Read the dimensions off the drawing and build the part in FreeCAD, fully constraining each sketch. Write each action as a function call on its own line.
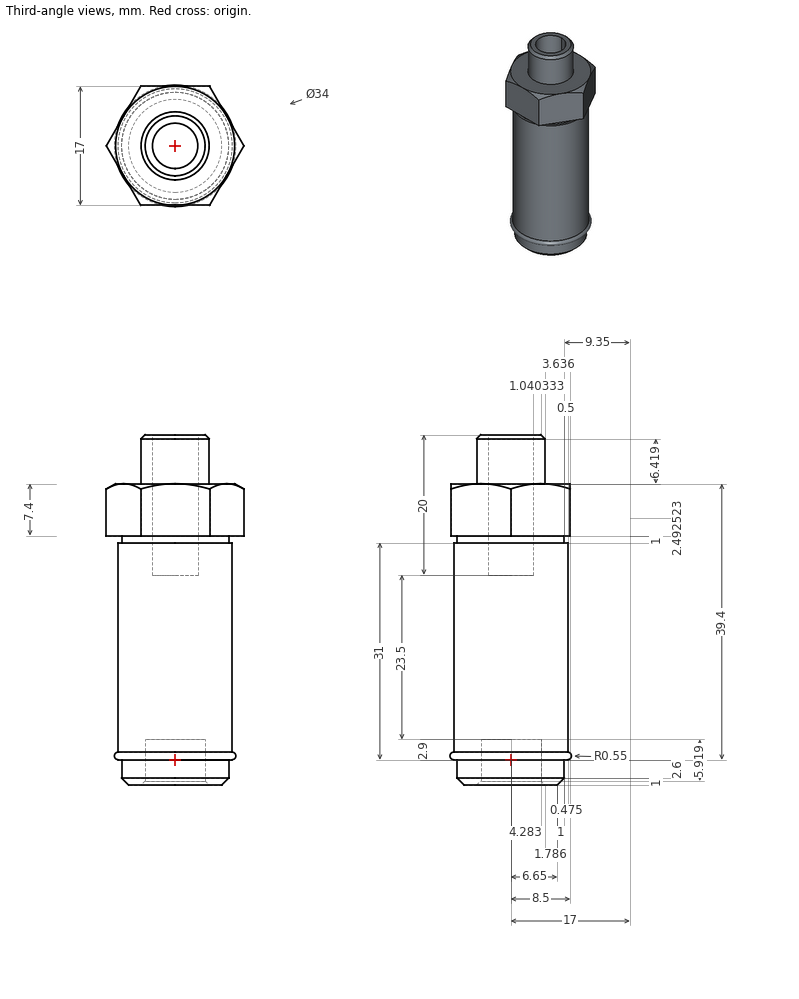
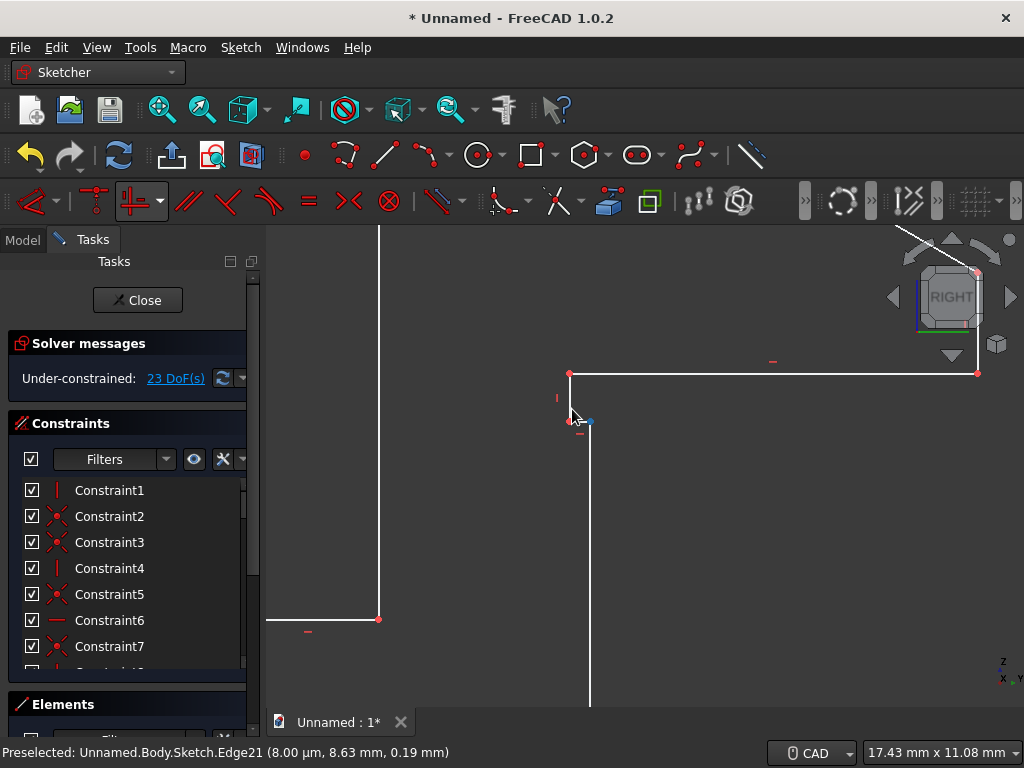
click(570, 407)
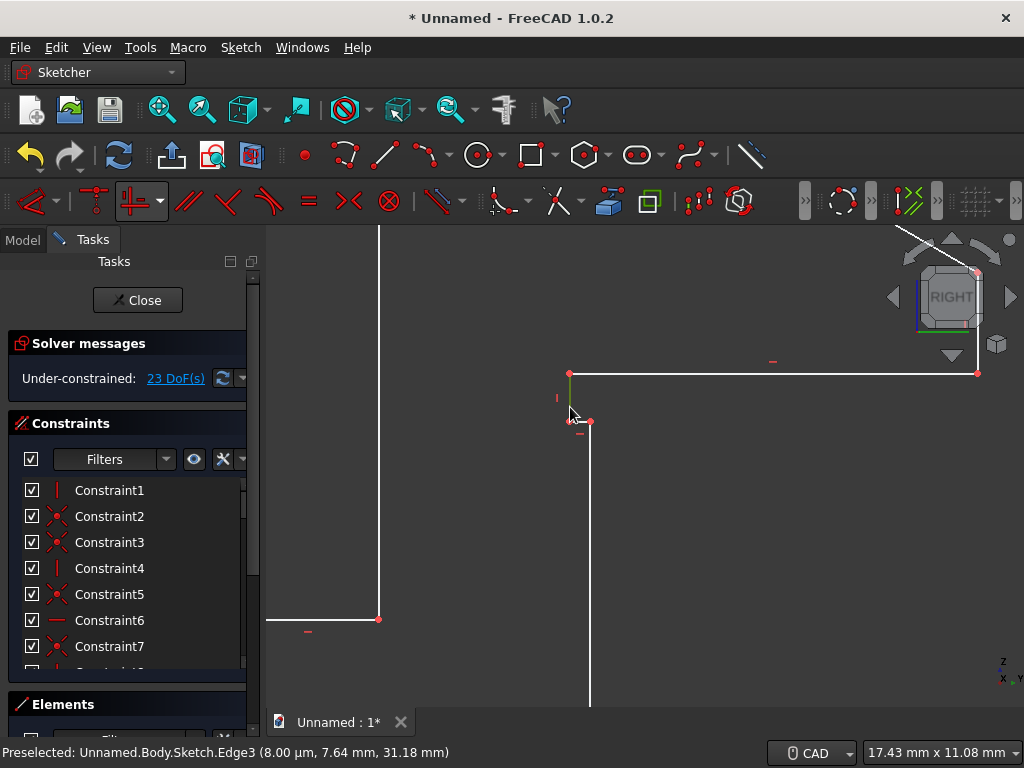
key(i)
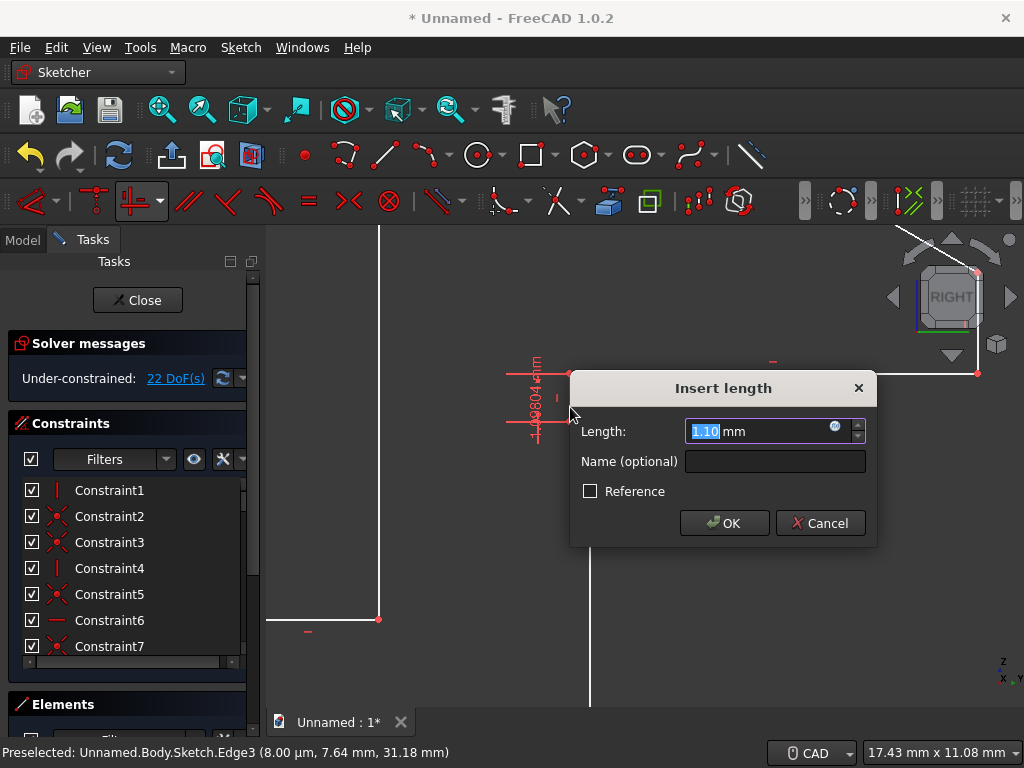
text(1)
key(Return)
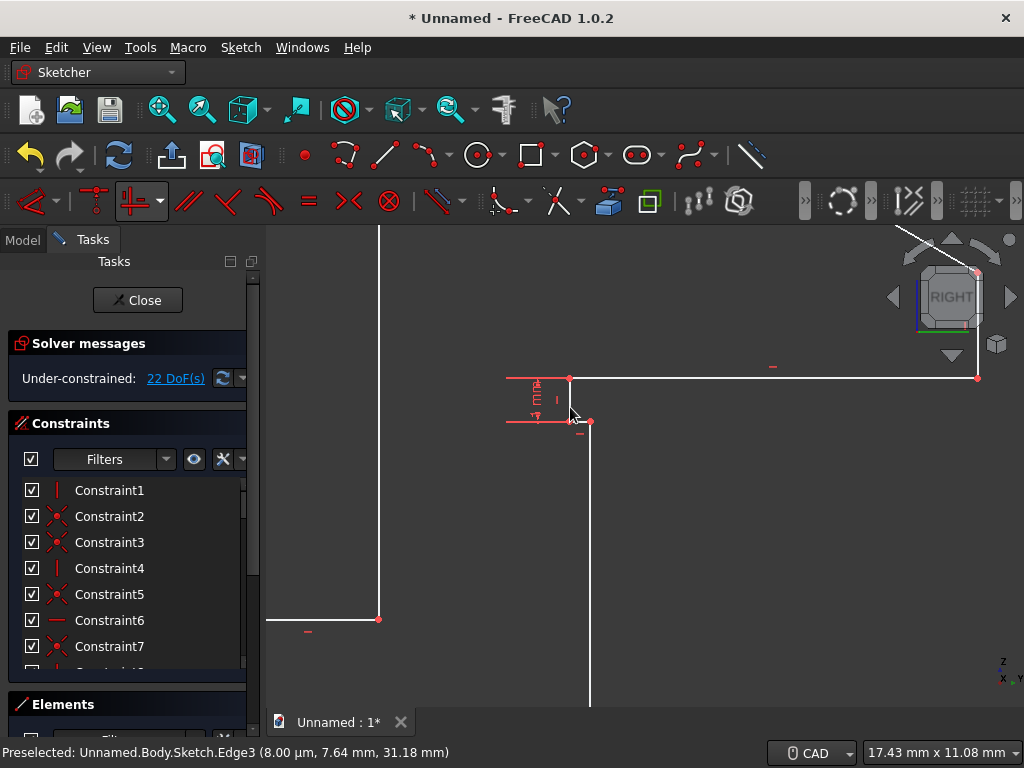
scroll(572, 408, down, 10)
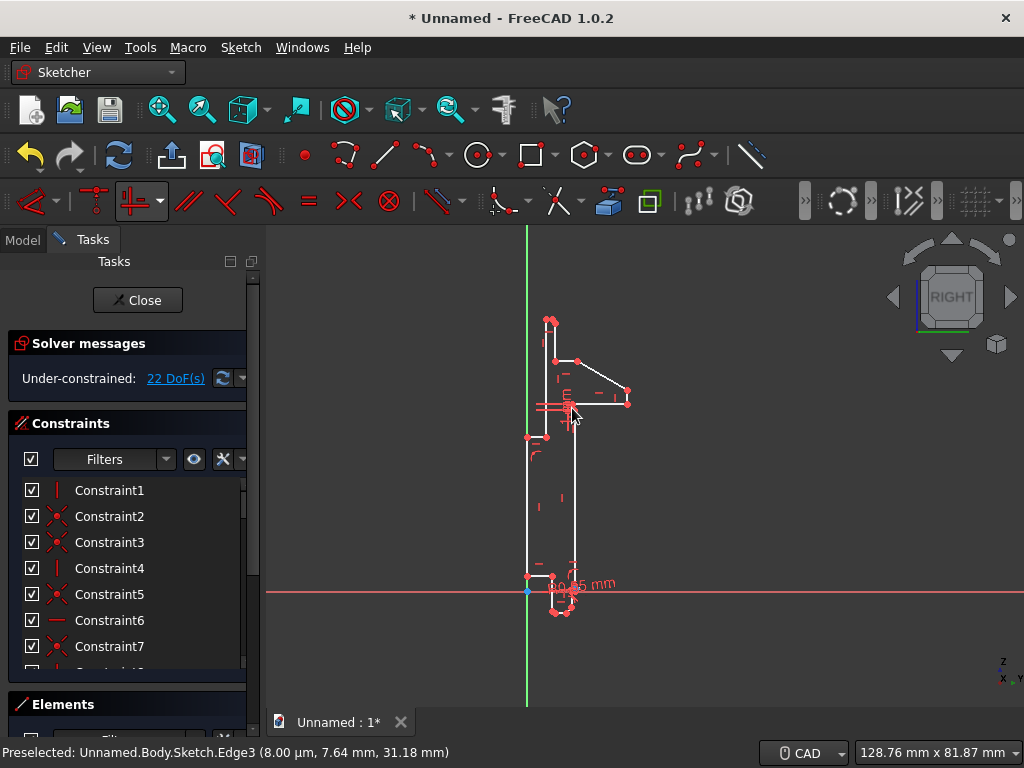
click(546, 402)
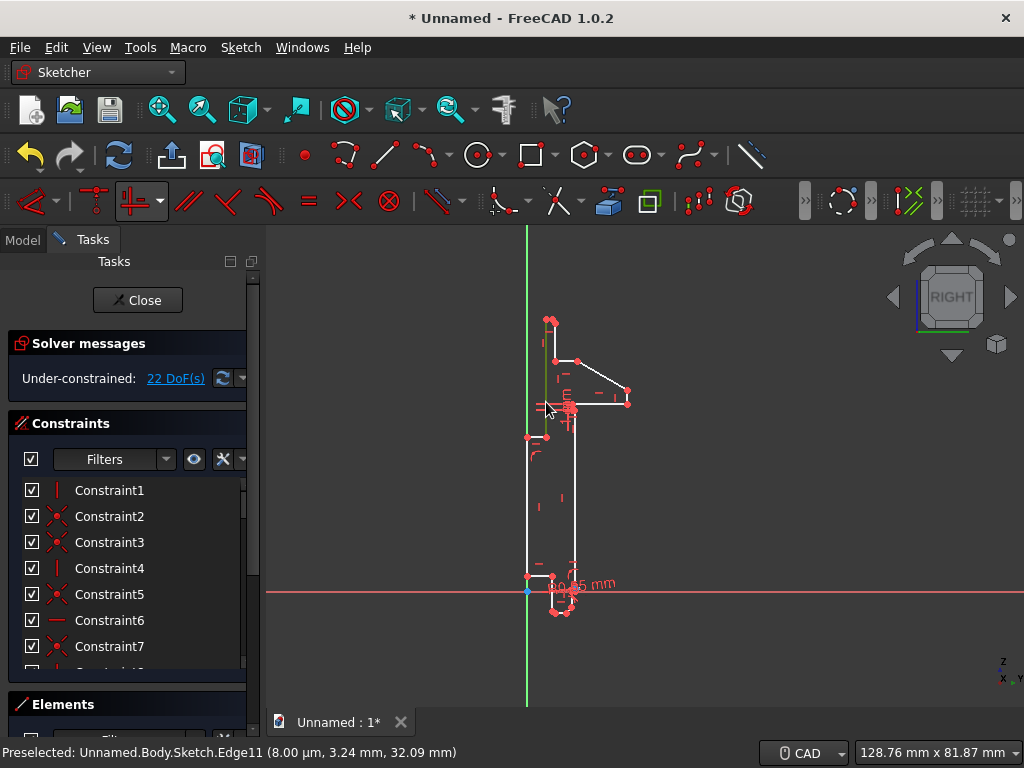
key(i)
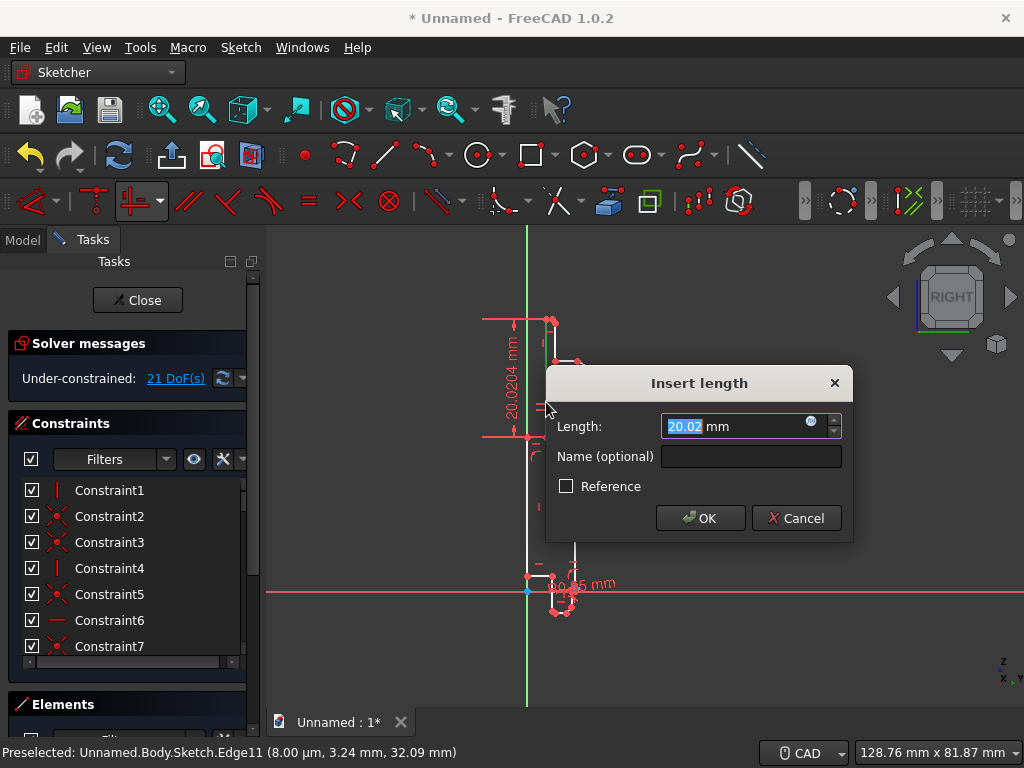
text(20)
key(Return)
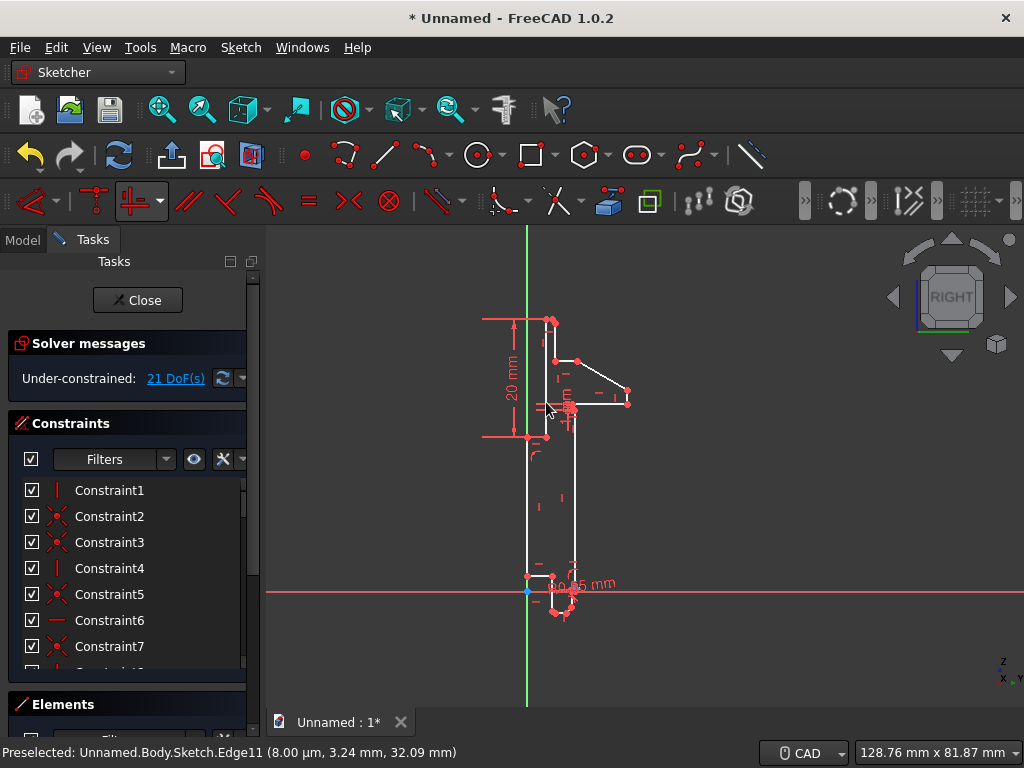
scroll(569, 610, up, 10)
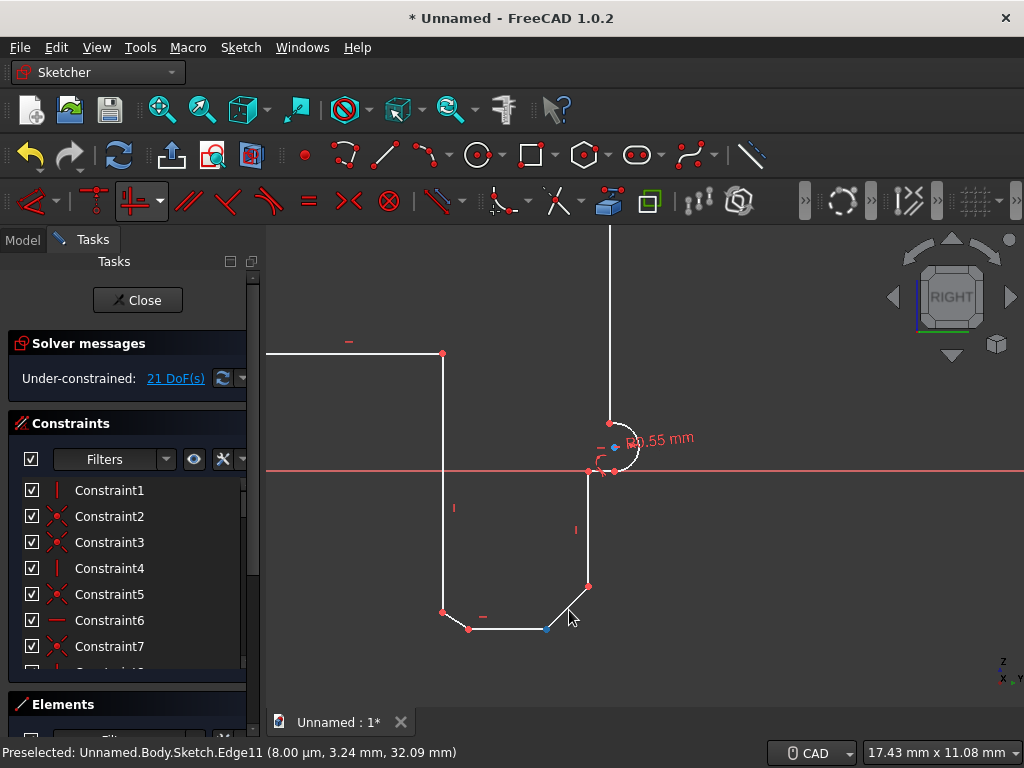
click(568, 608)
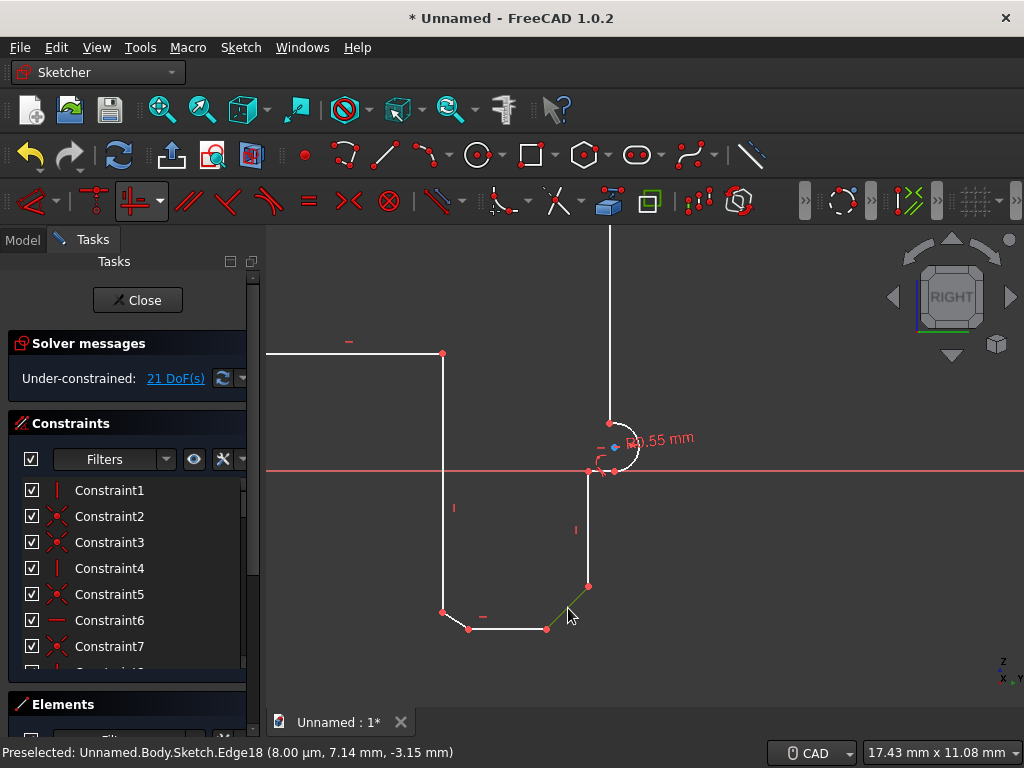
key(l)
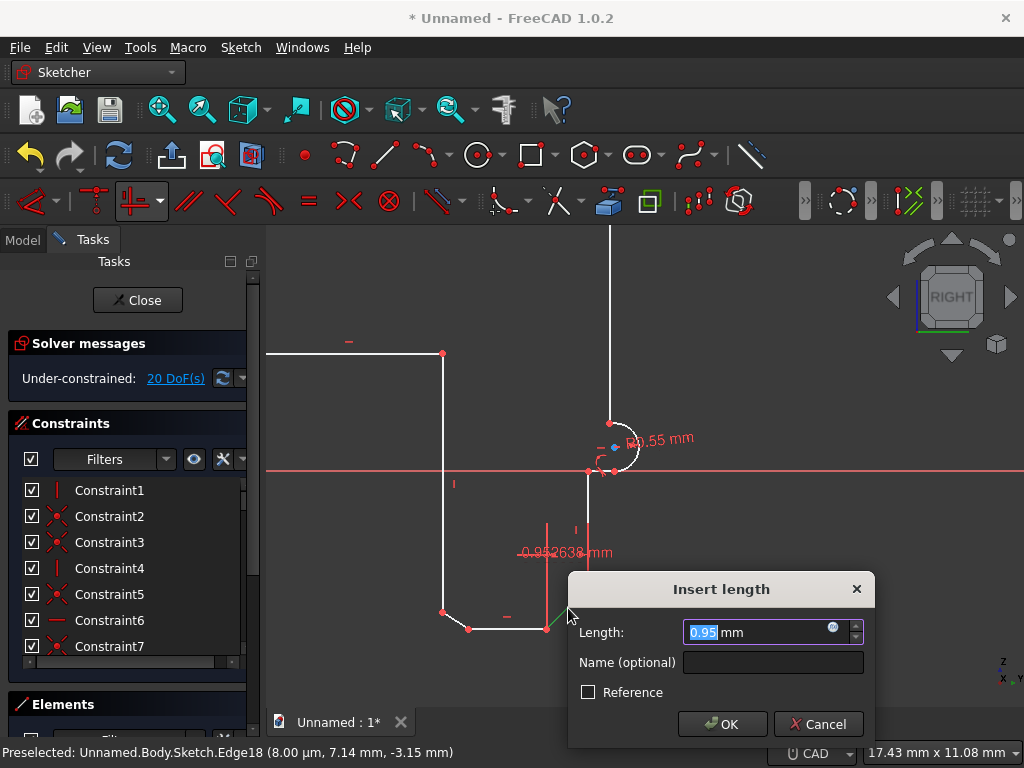
text(1)
key(Return)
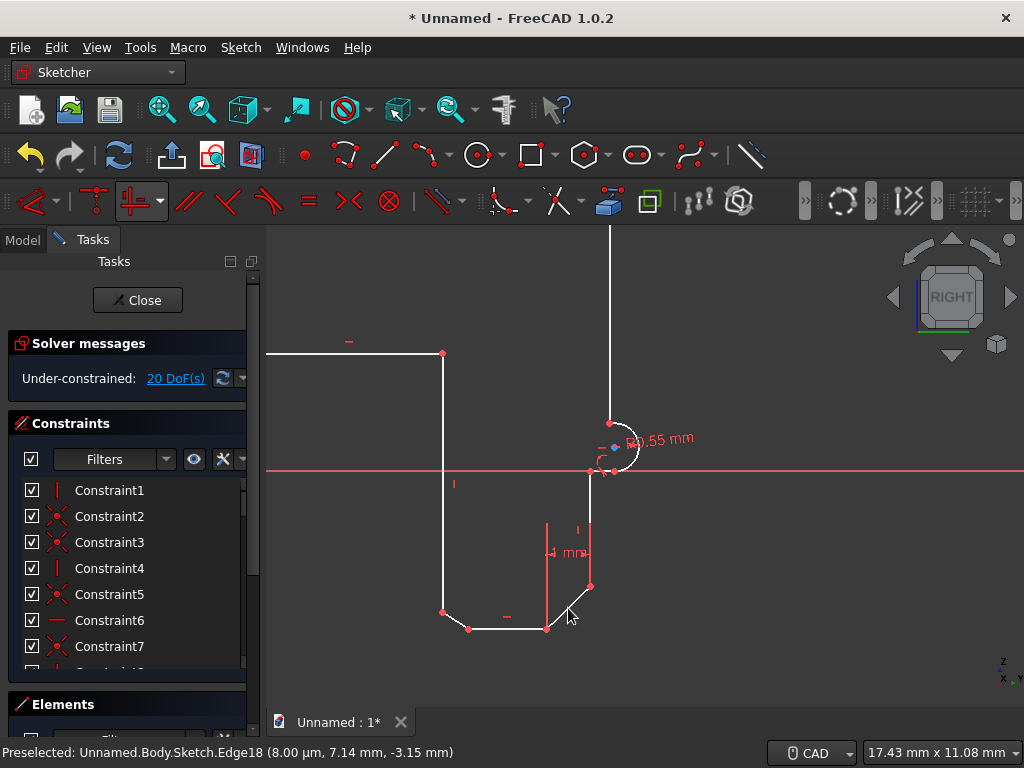
click(560, 616)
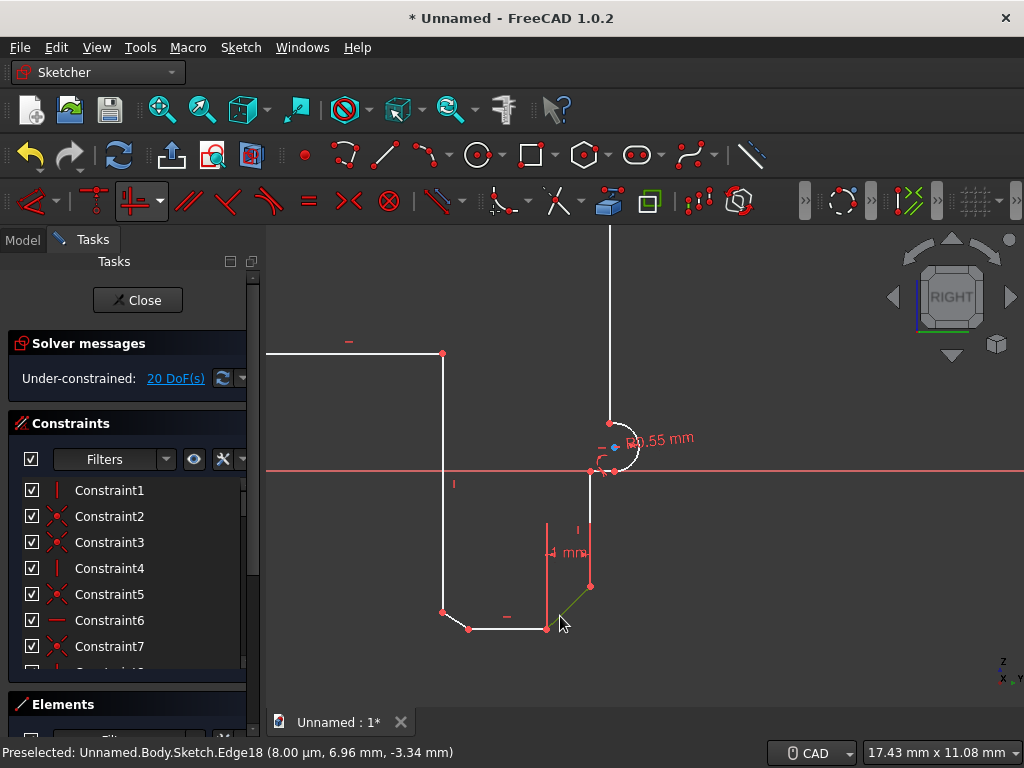
click(58, 202)